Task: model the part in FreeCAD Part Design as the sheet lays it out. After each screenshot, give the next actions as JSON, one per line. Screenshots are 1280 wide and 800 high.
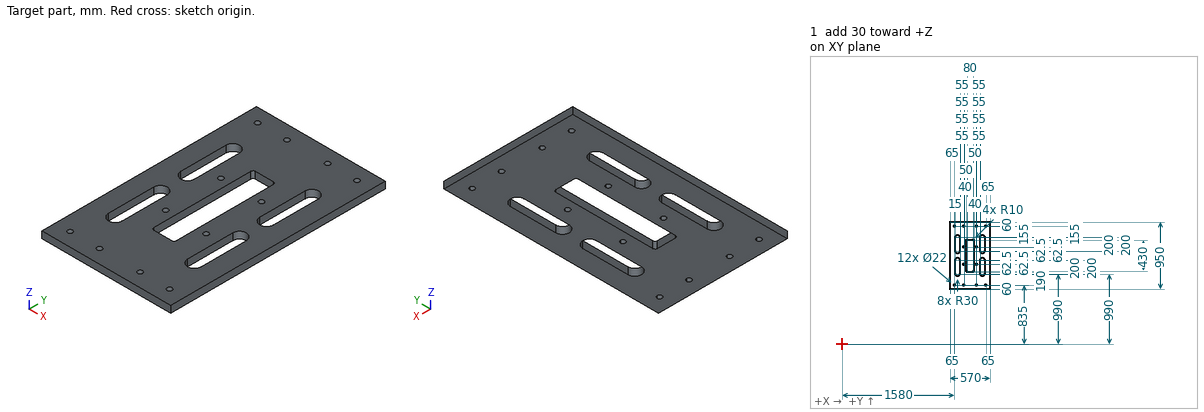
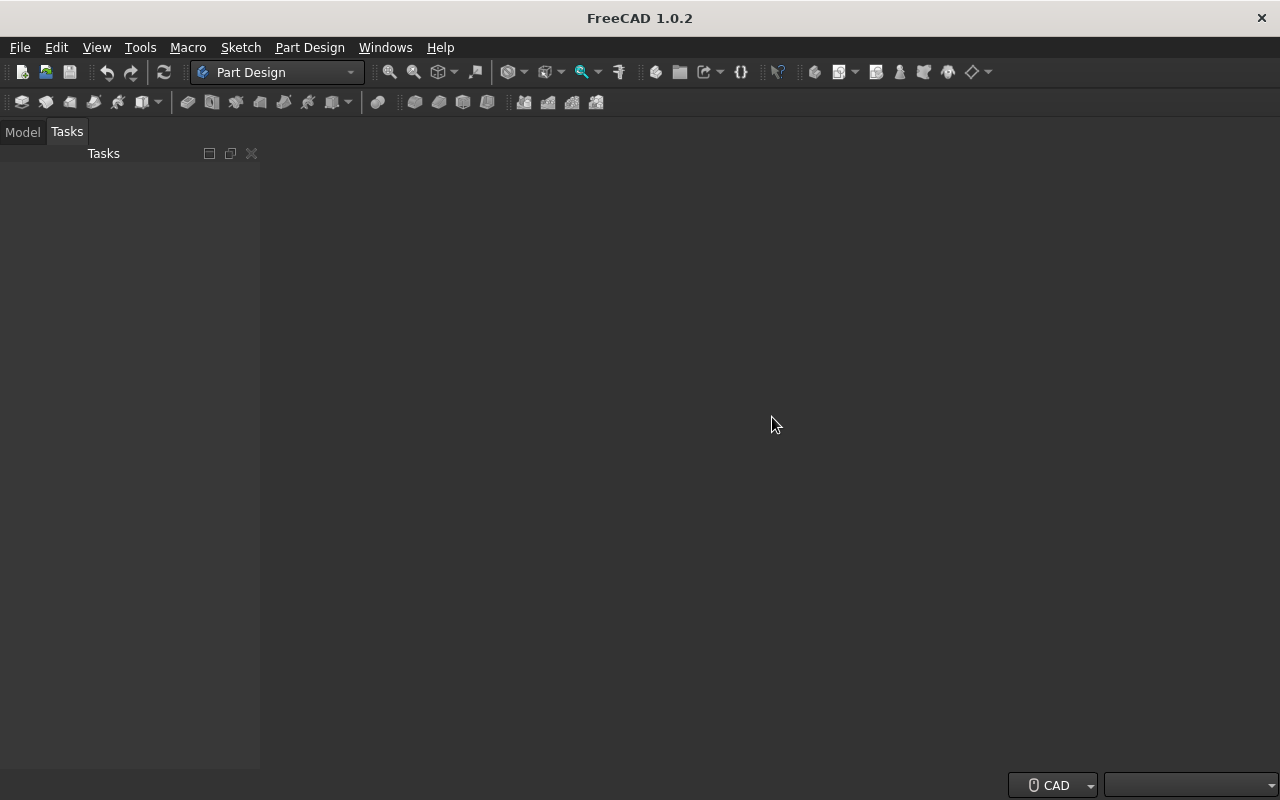
{"action": "left_click", "coordinate": [22, 72]}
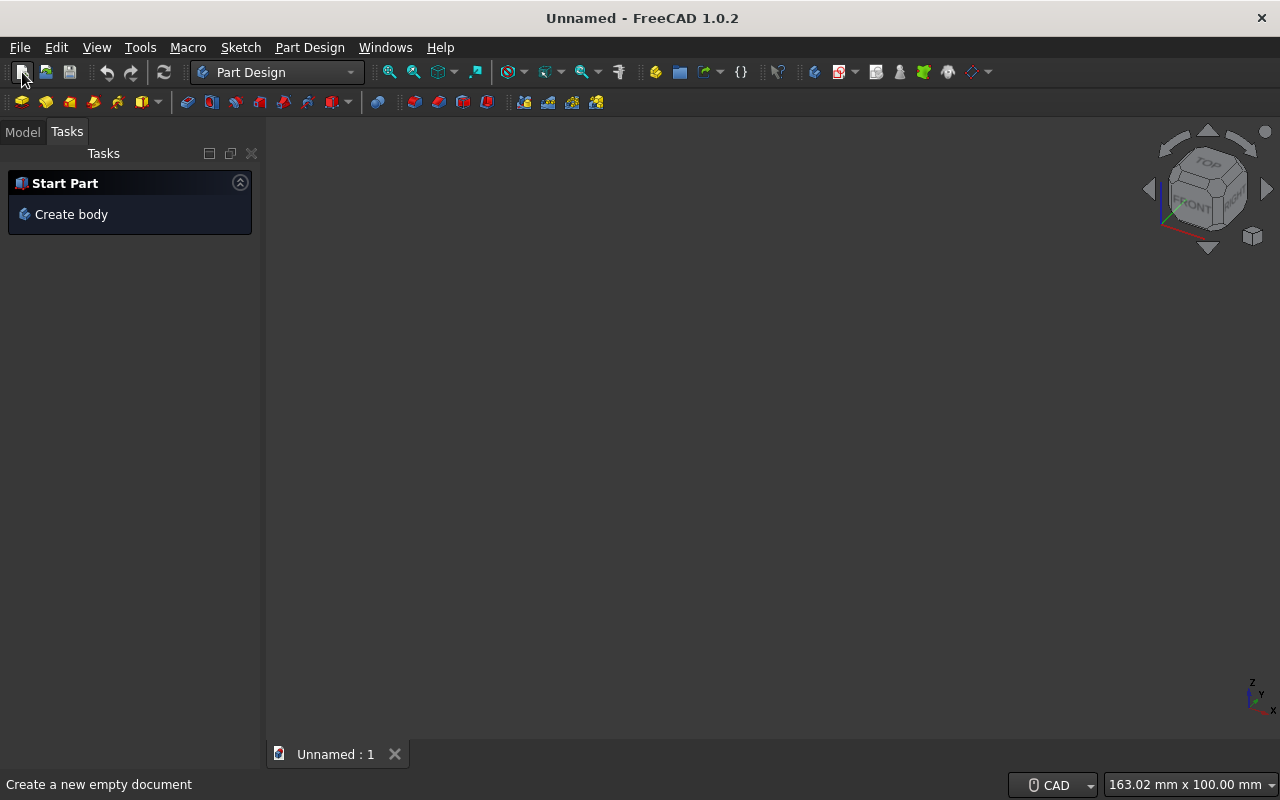
{"action": "left_click", "coordinate": [840, 72]}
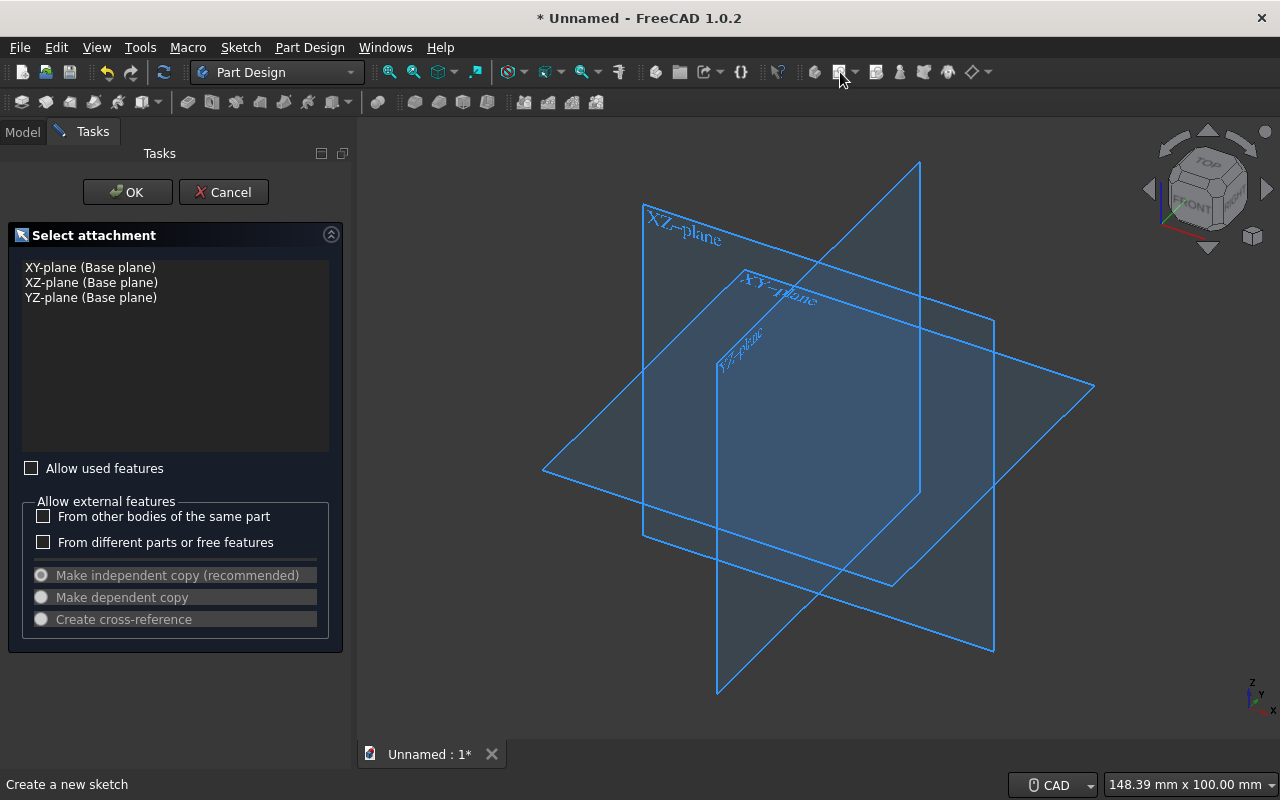
{"action": "left_click", "coordinate": [82, 268]}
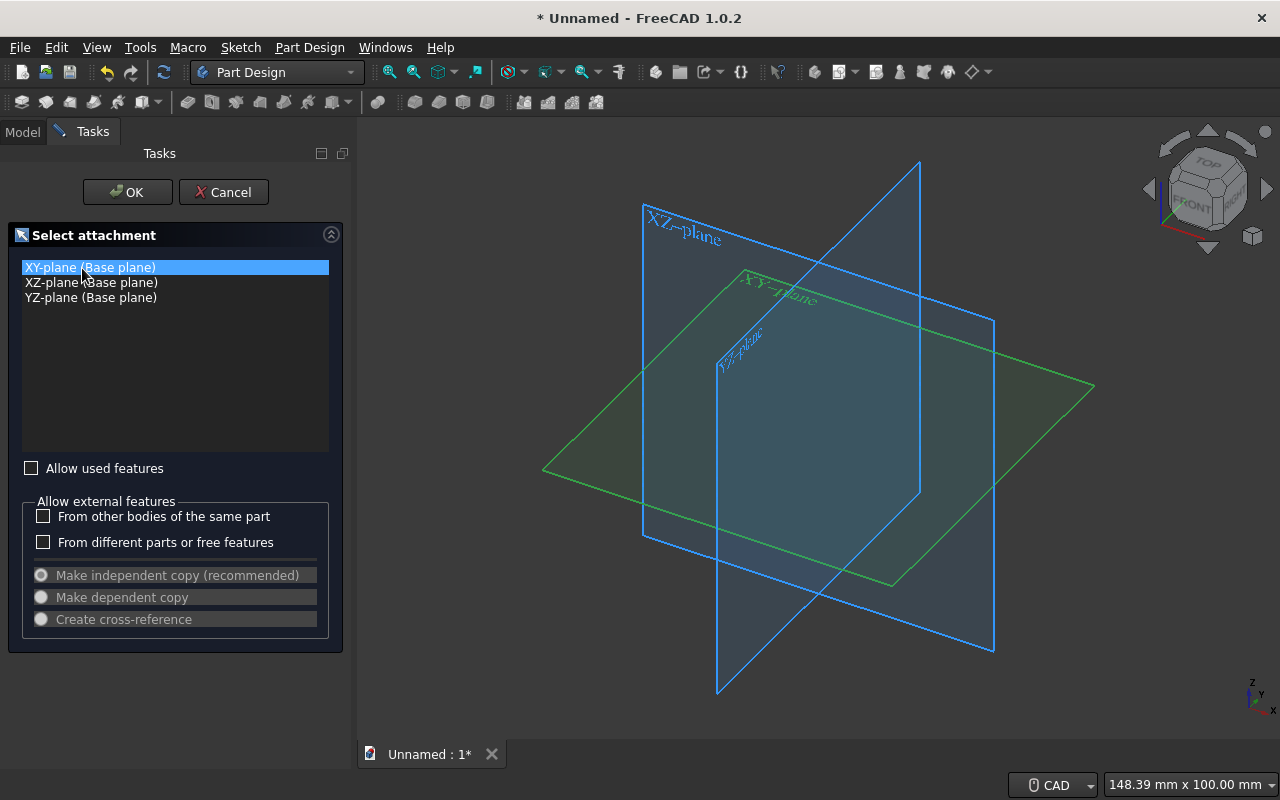
{"action": "left_click", "coordinate": [128, 192]}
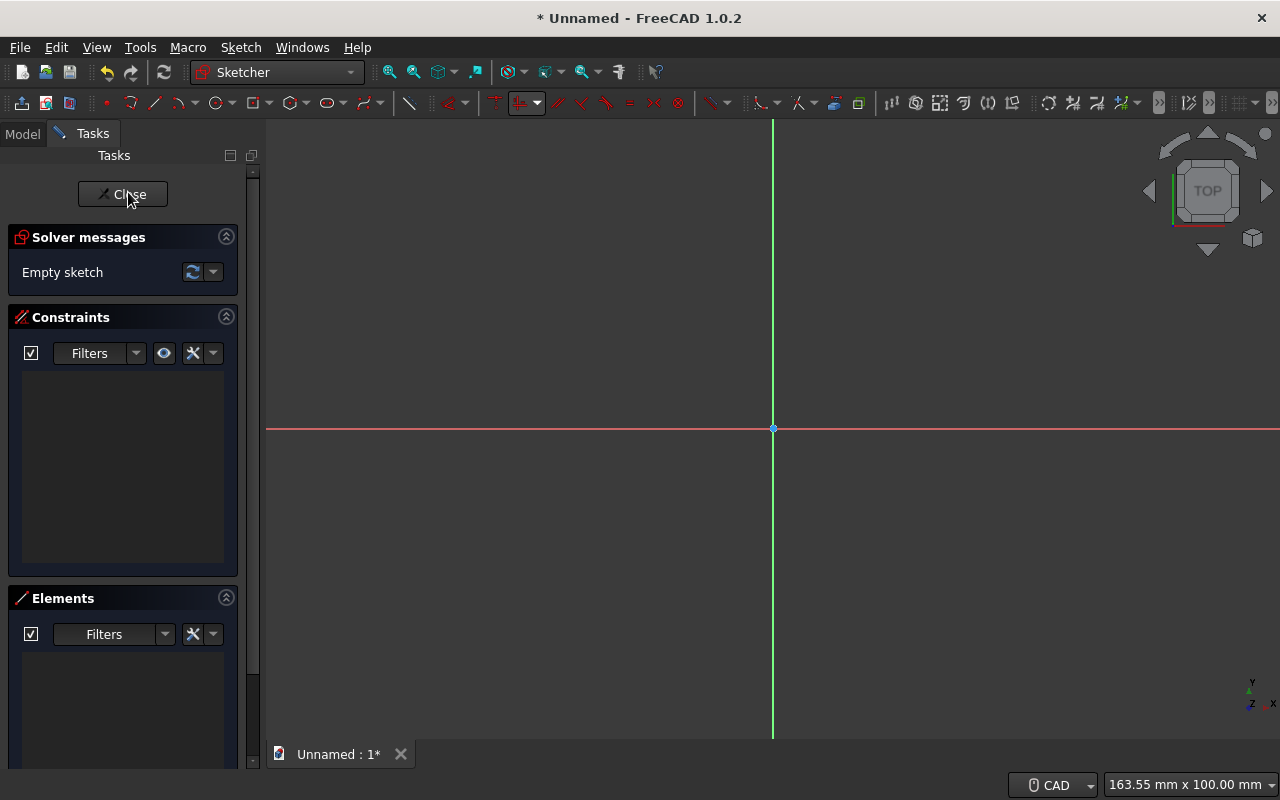
{"action": "scroll", "coordinate": [427, 656], "scroll_direction": "down", "scroll_amount": 16}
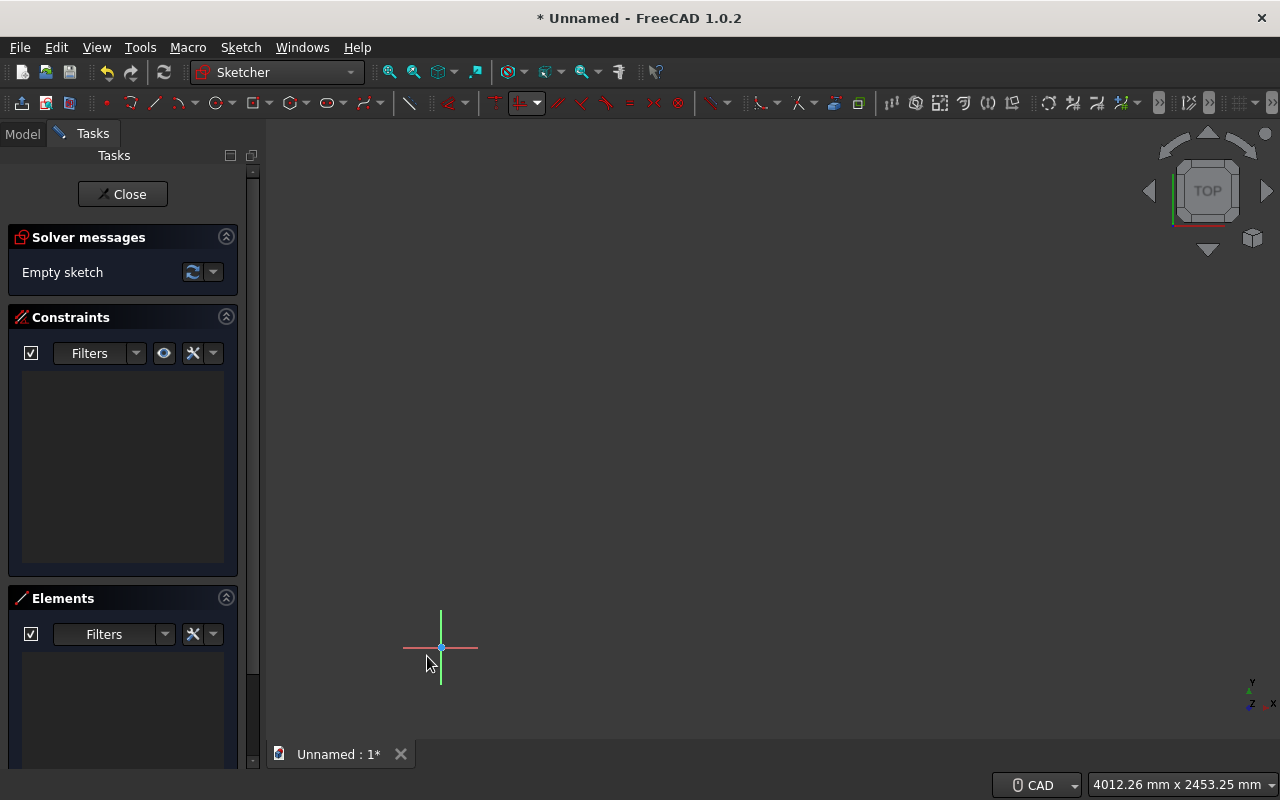
{"action": "key", "text": "g r"}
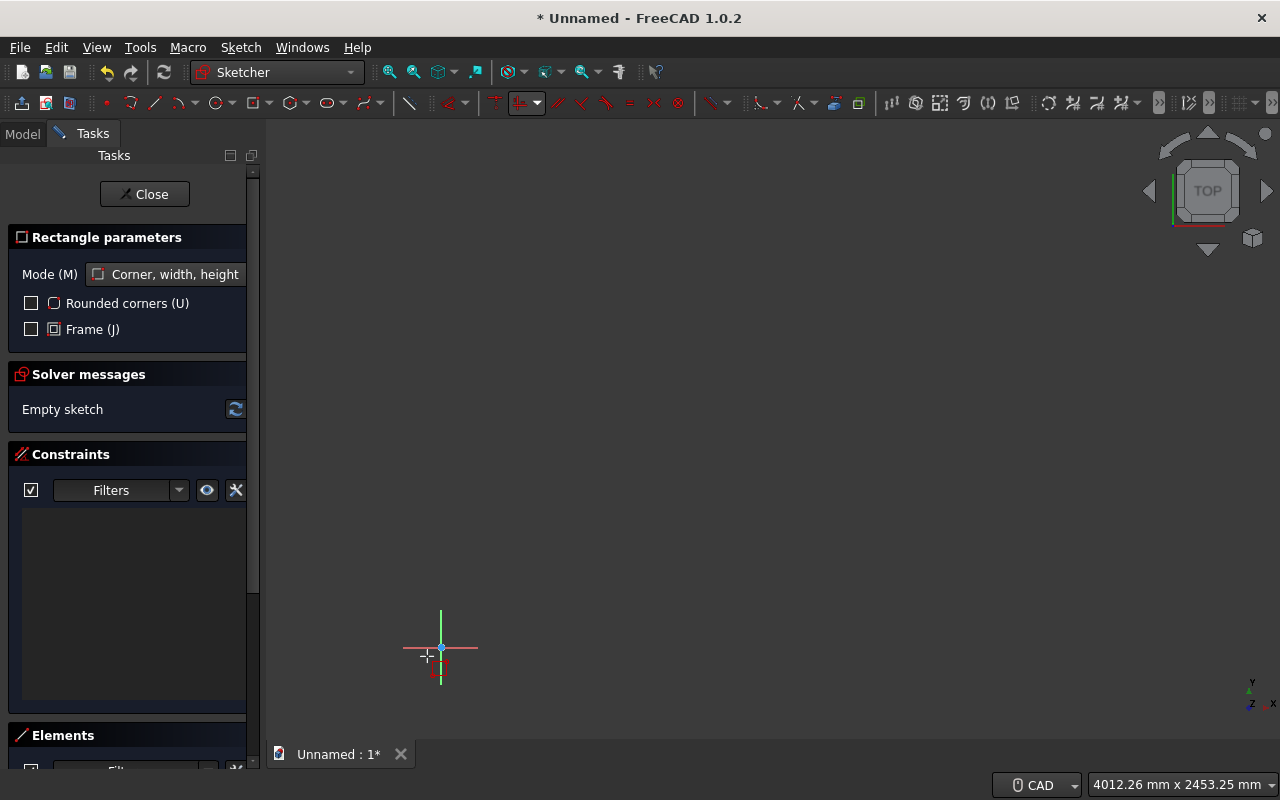
{"action": "left_click", "coordinate": [824, 212]}
{"action": "left_click", "coordinate": [968, 452]}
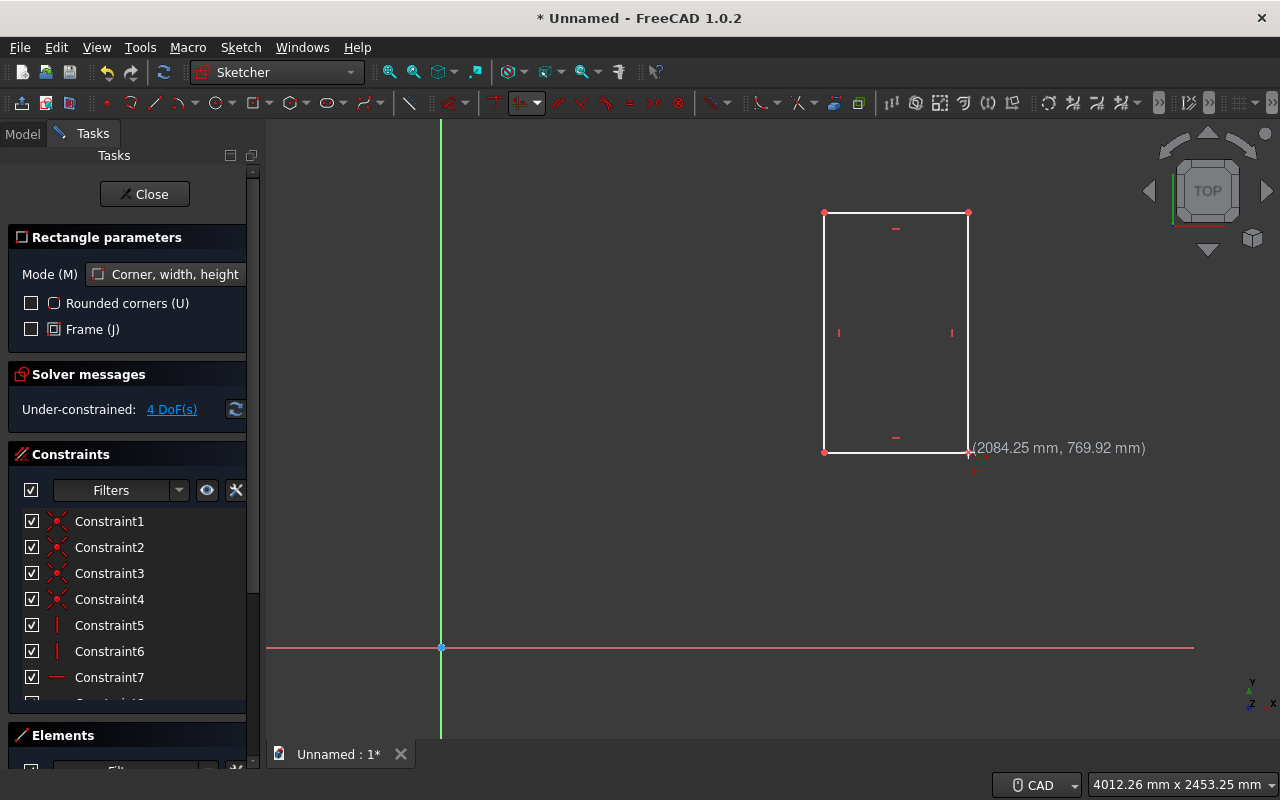
{"action": "left_click", "coordinate": [328, 104]}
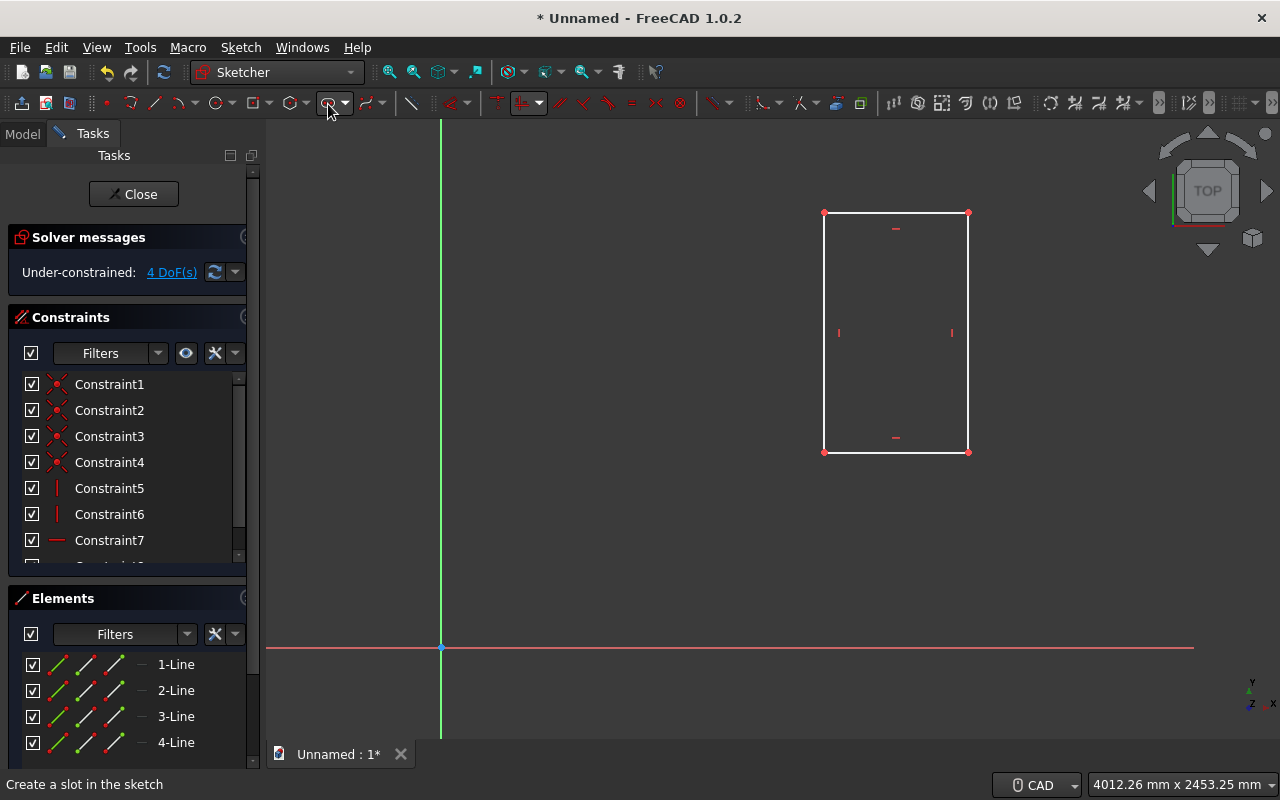
{"action": "scroll", "coordinate": [852, 397], "scroll_direction": "up", "scroll_amount": 6}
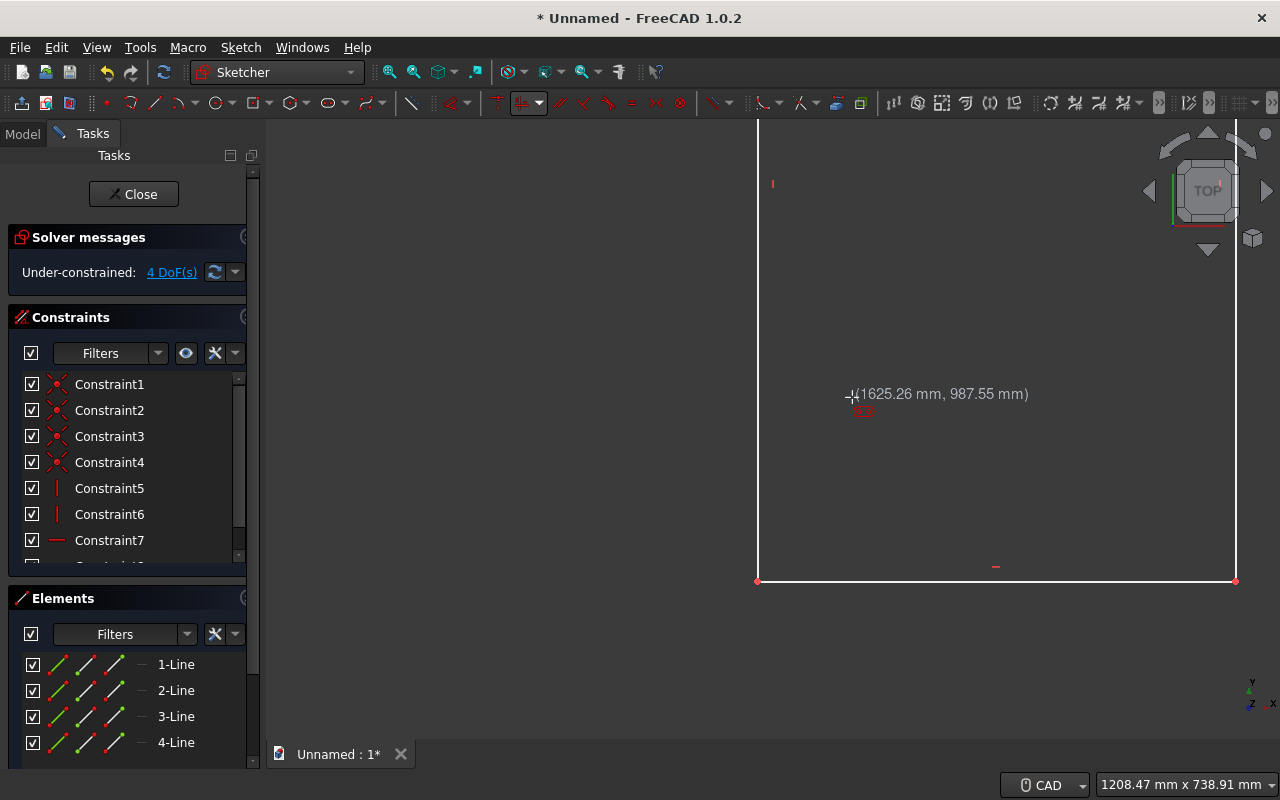
{"action": "left_click", "coordinate": [850, 397]}